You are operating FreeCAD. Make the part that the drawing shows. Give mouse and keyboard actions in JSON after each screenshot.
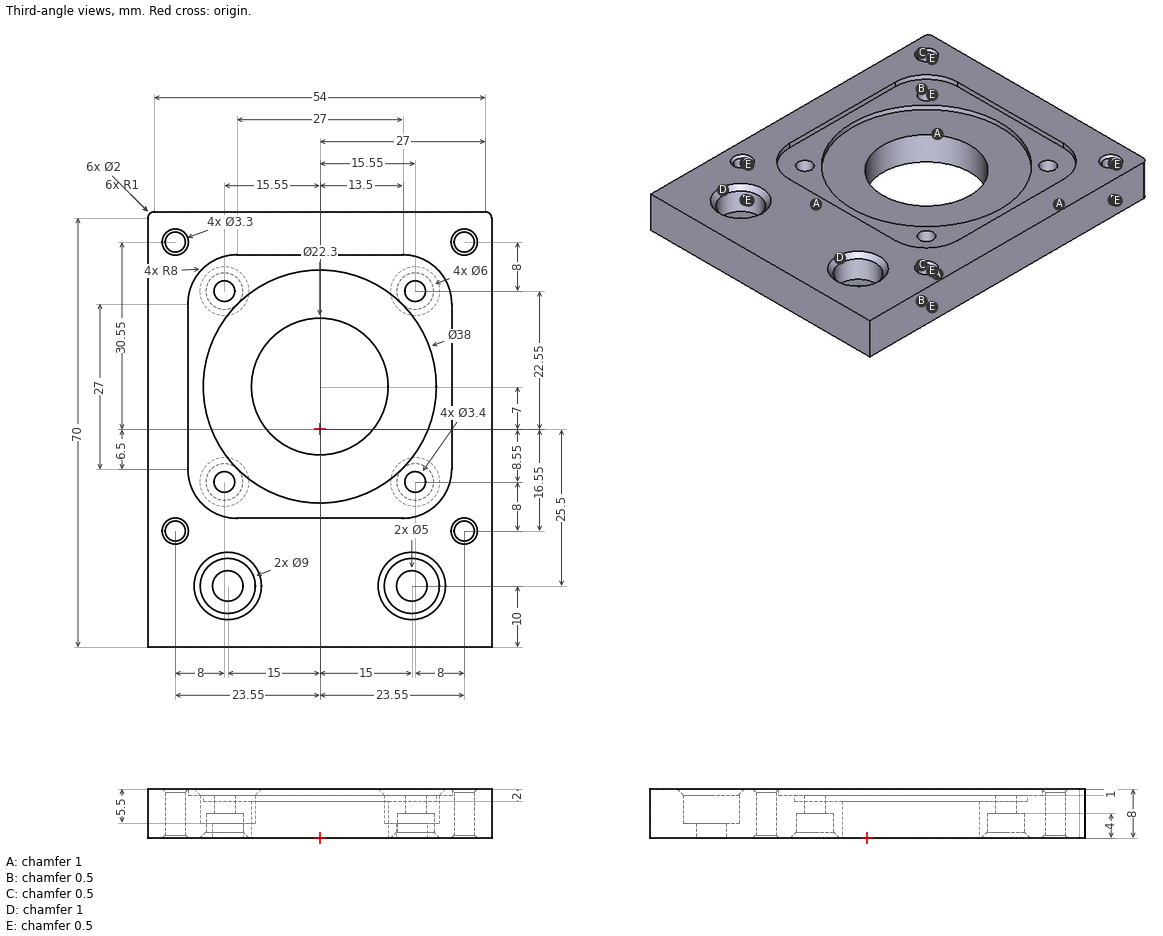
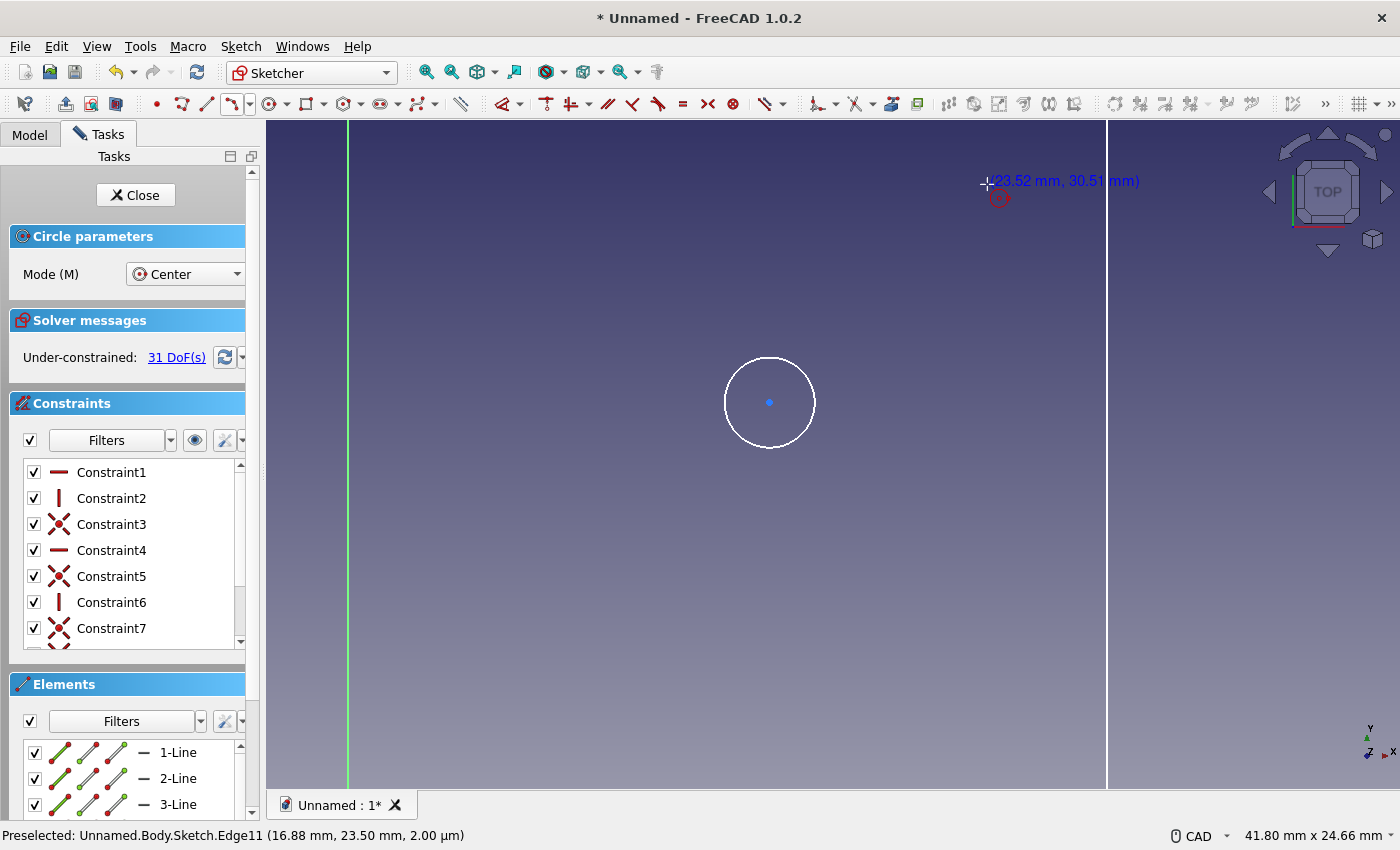
{"action": "scroll", "coordinate": [901, 272], "scroll_direction": "down", "scroll_amount": 7}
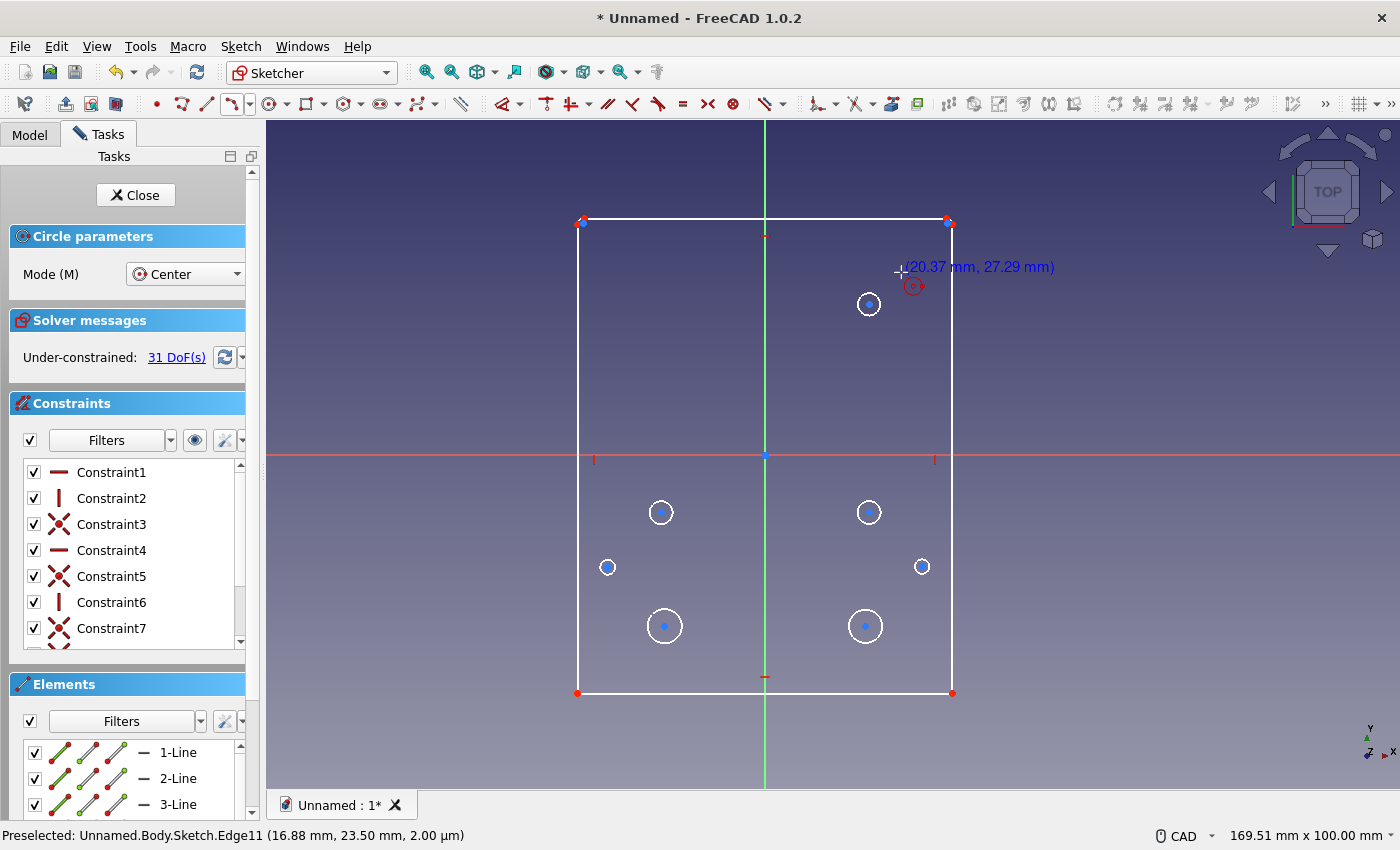
{"action": "left_click", "coordinate": [923, 251]}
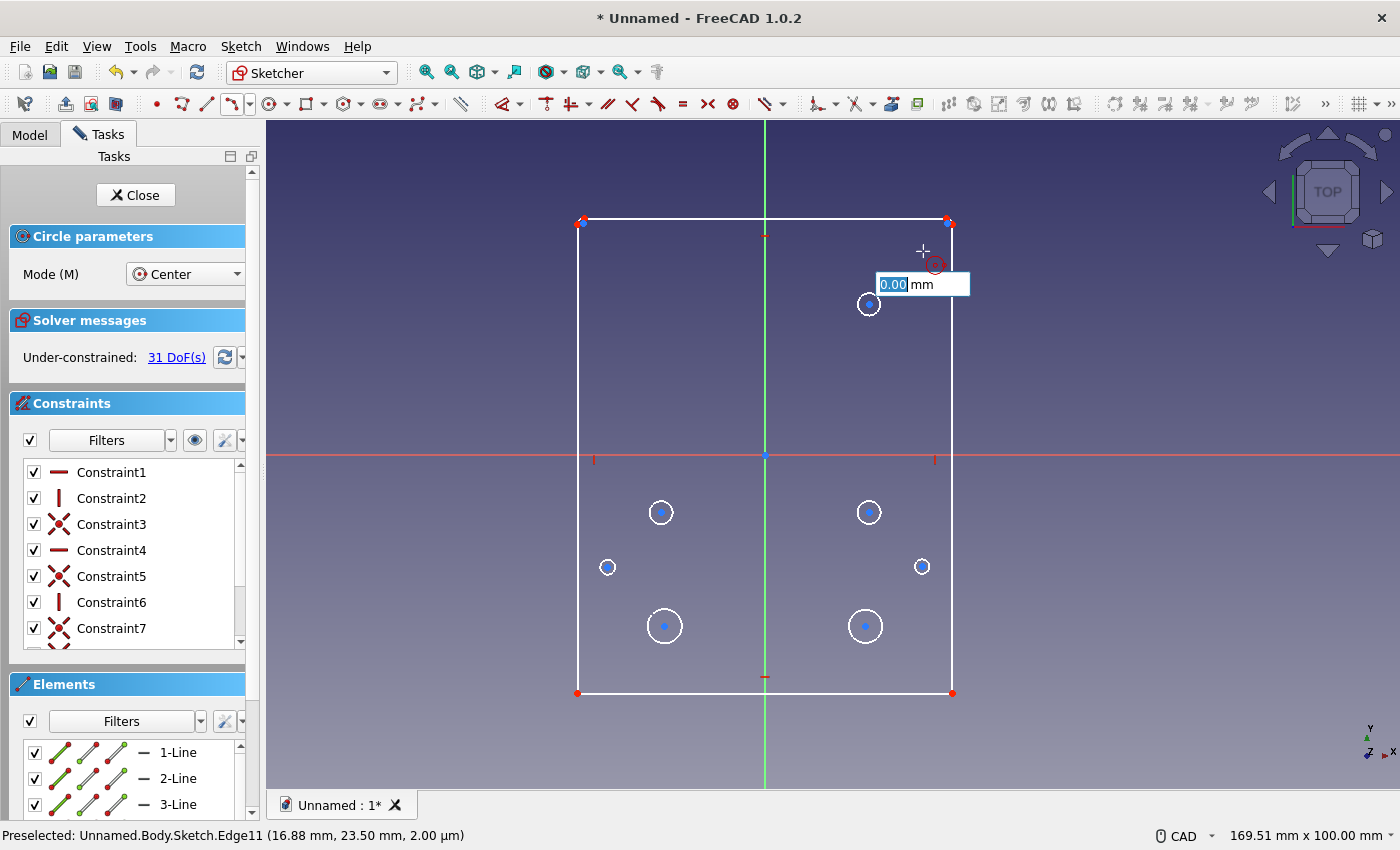
{"action": "scroll", "coordinate": [927, 246], "scroll_direction": "up", "scroll_amount": 5}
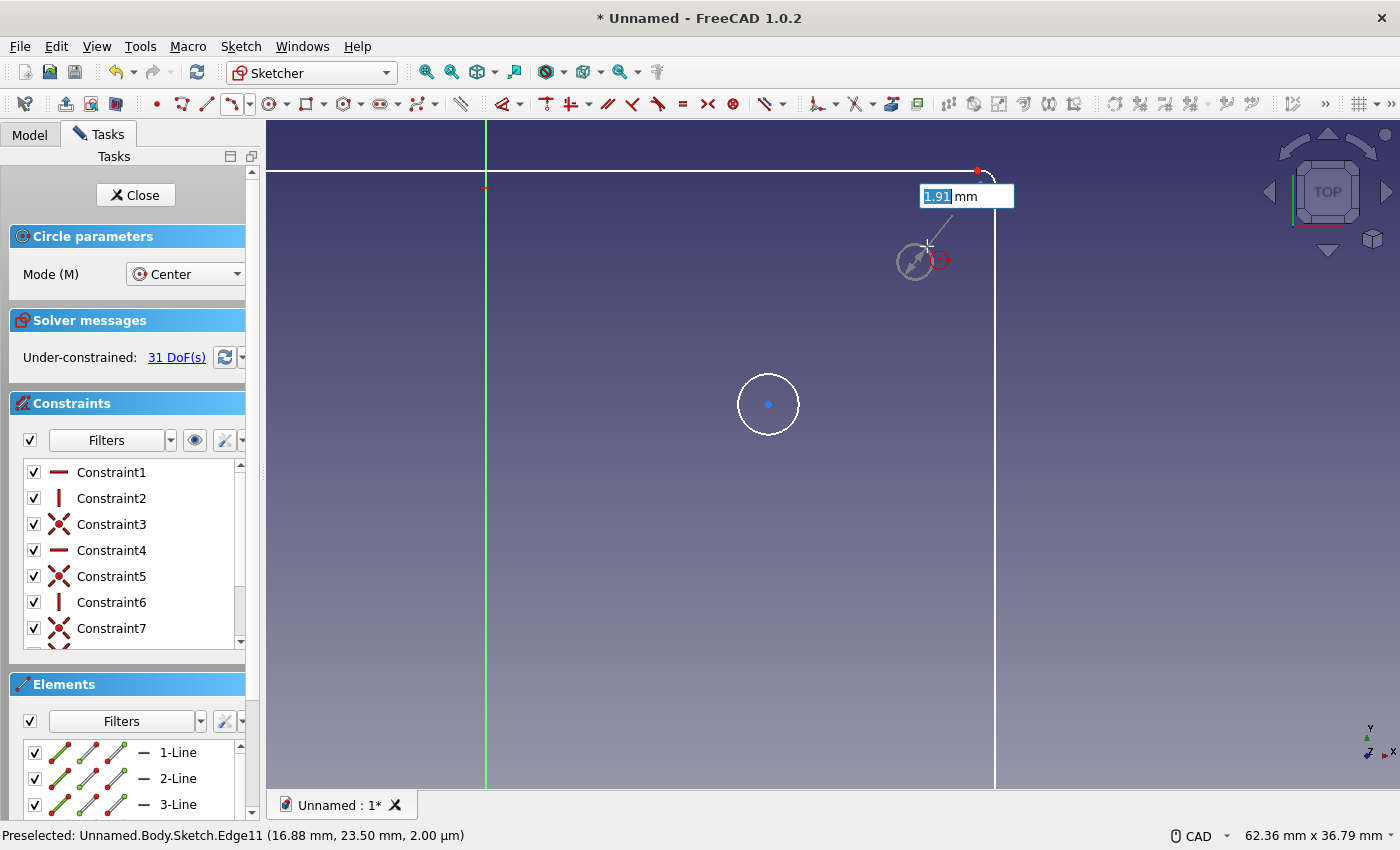
{"action": "left_click", "coordinate": [927, 245]}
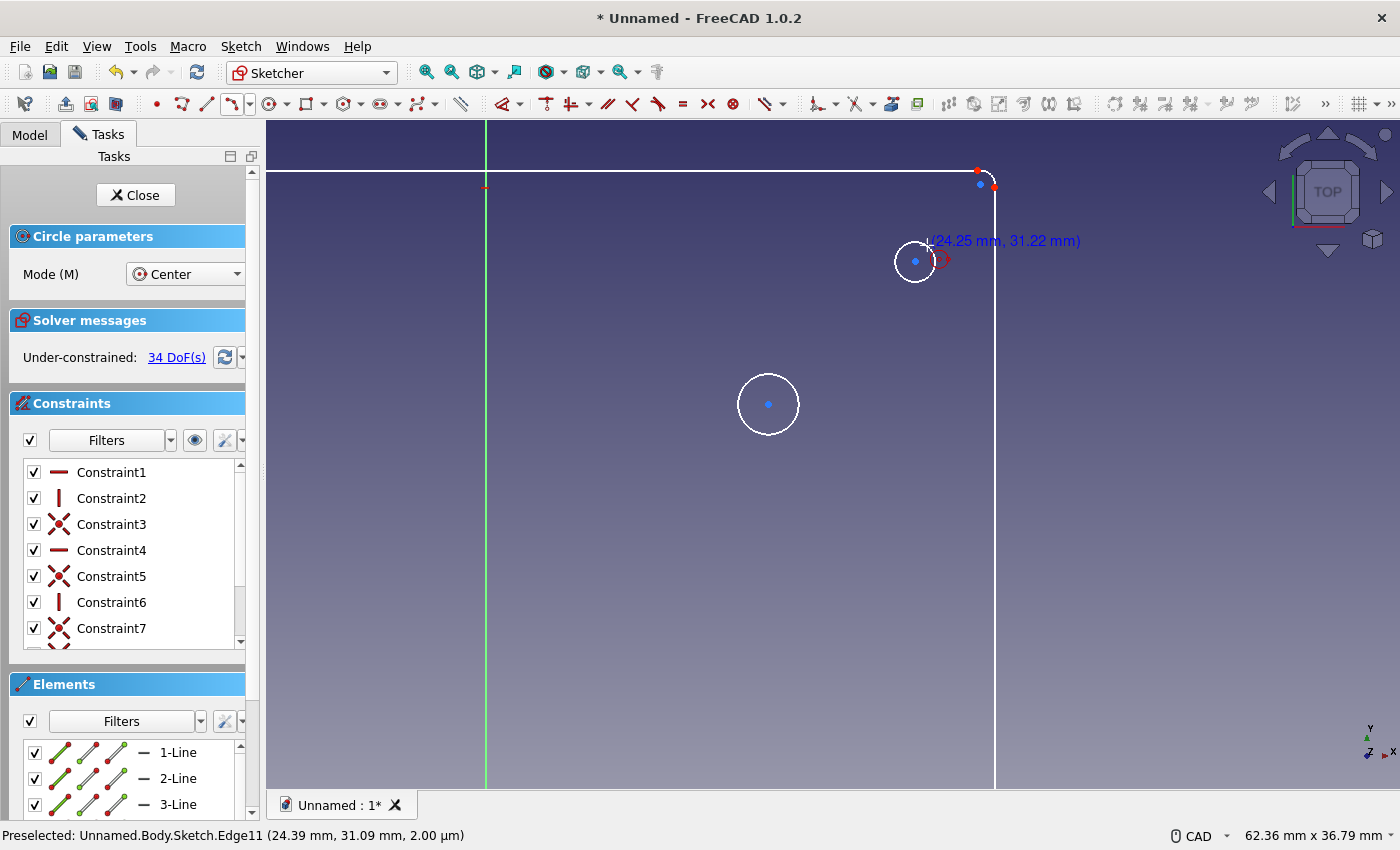
{"action": "left_click", "coordinate": [486, 687]}
{"action": "left_click", "coordinate": [629, 543]}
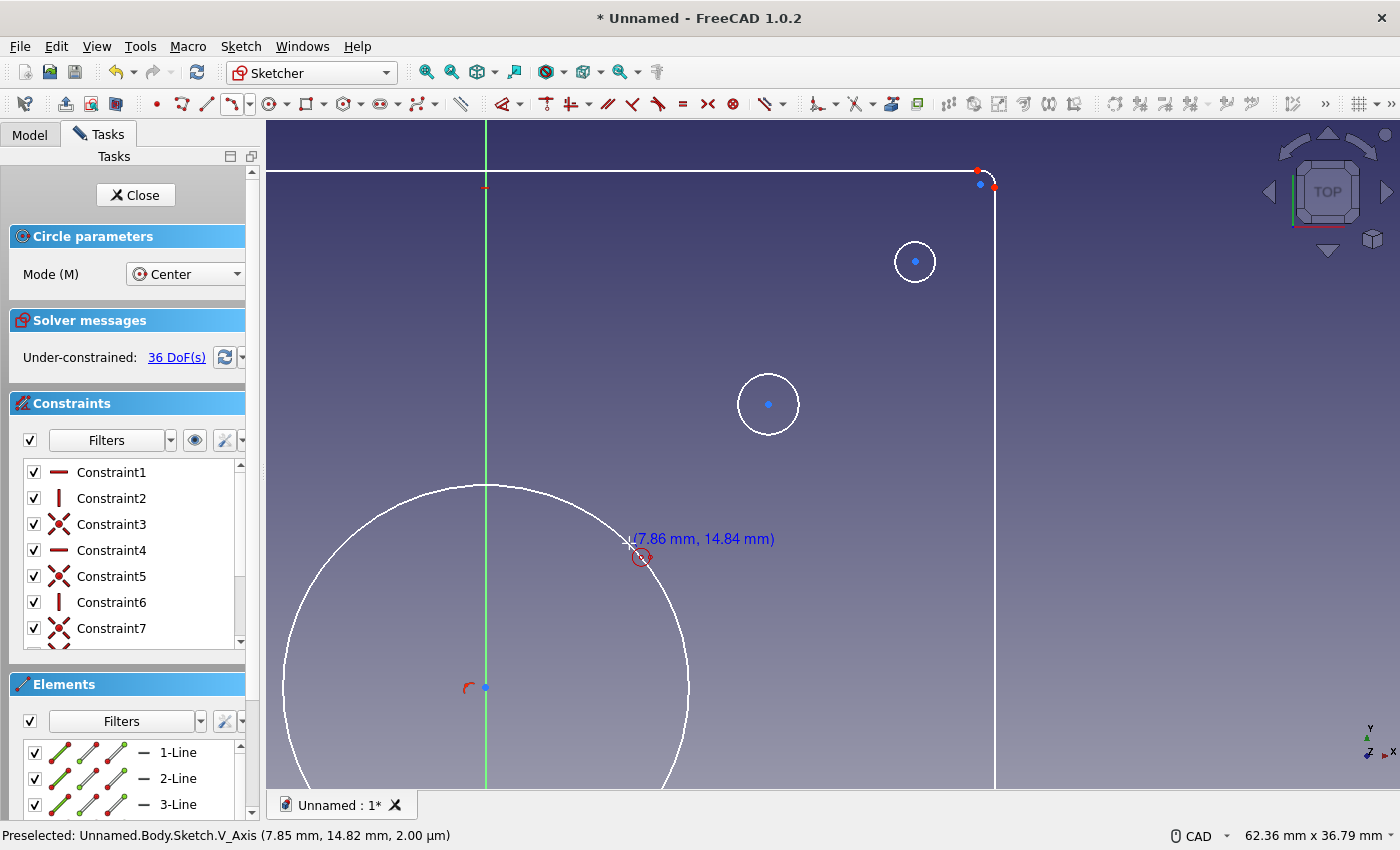
{"action": "scroll", "coordinate": [927, 245], "scroll_direction": "down", "scroll_amount": 5}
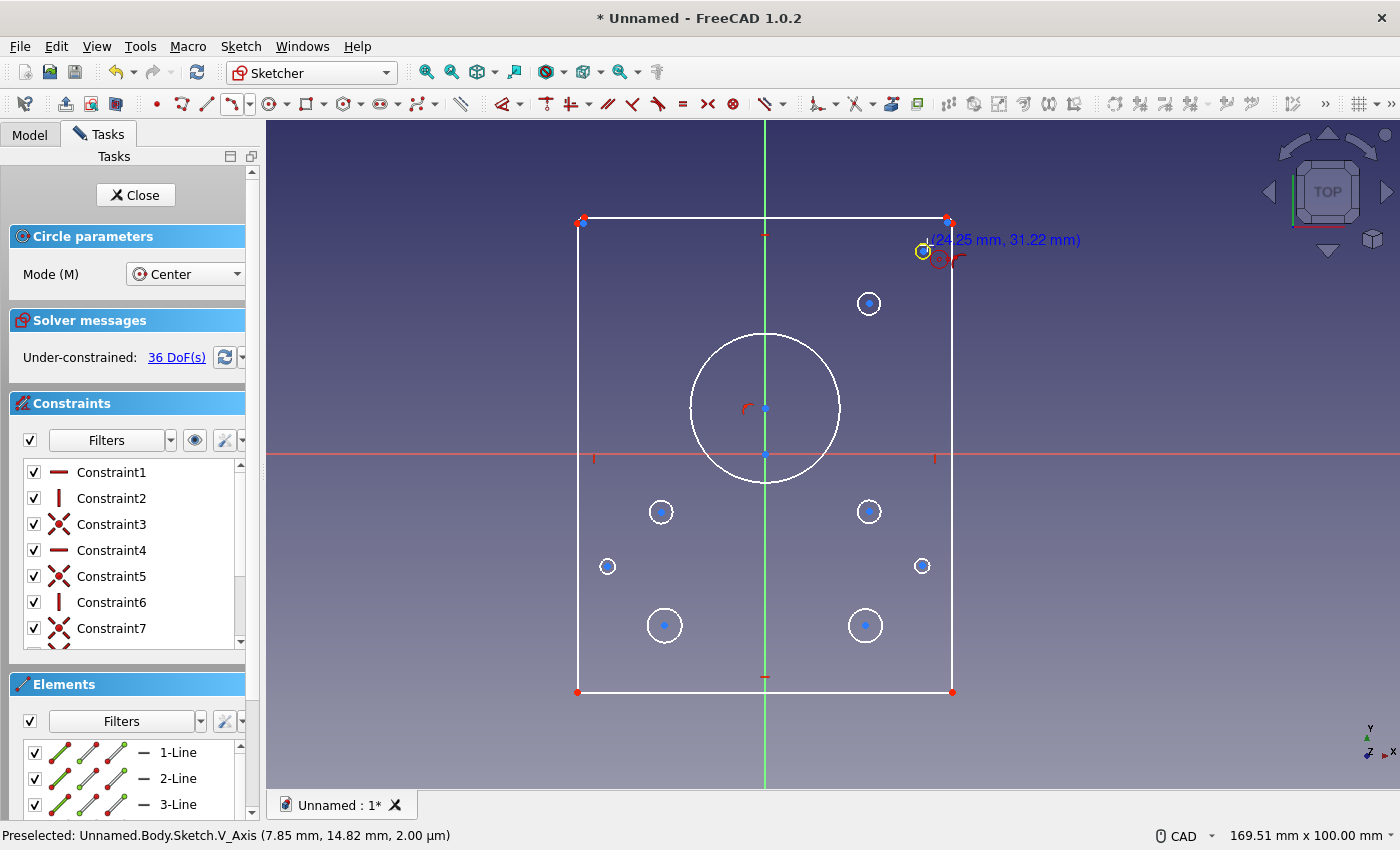
{"action": "scroll", "coordinate": [661, 304], "scroll_direction": "up", "scroll_amount": 4}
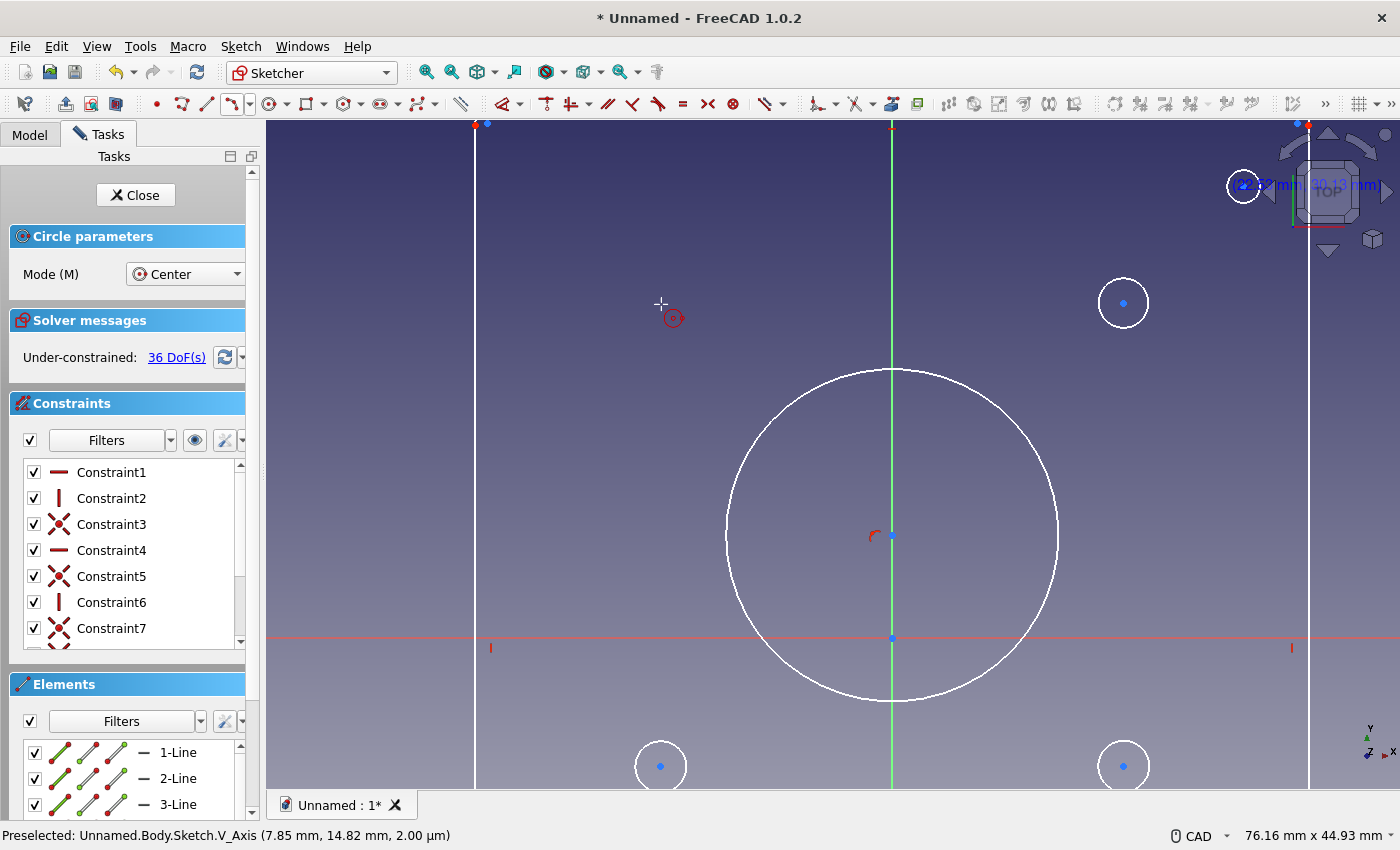
{"action": "left_click", "coordinate": [661, 303]}
{"action": "left_click", "coordinate": [679, 285]}